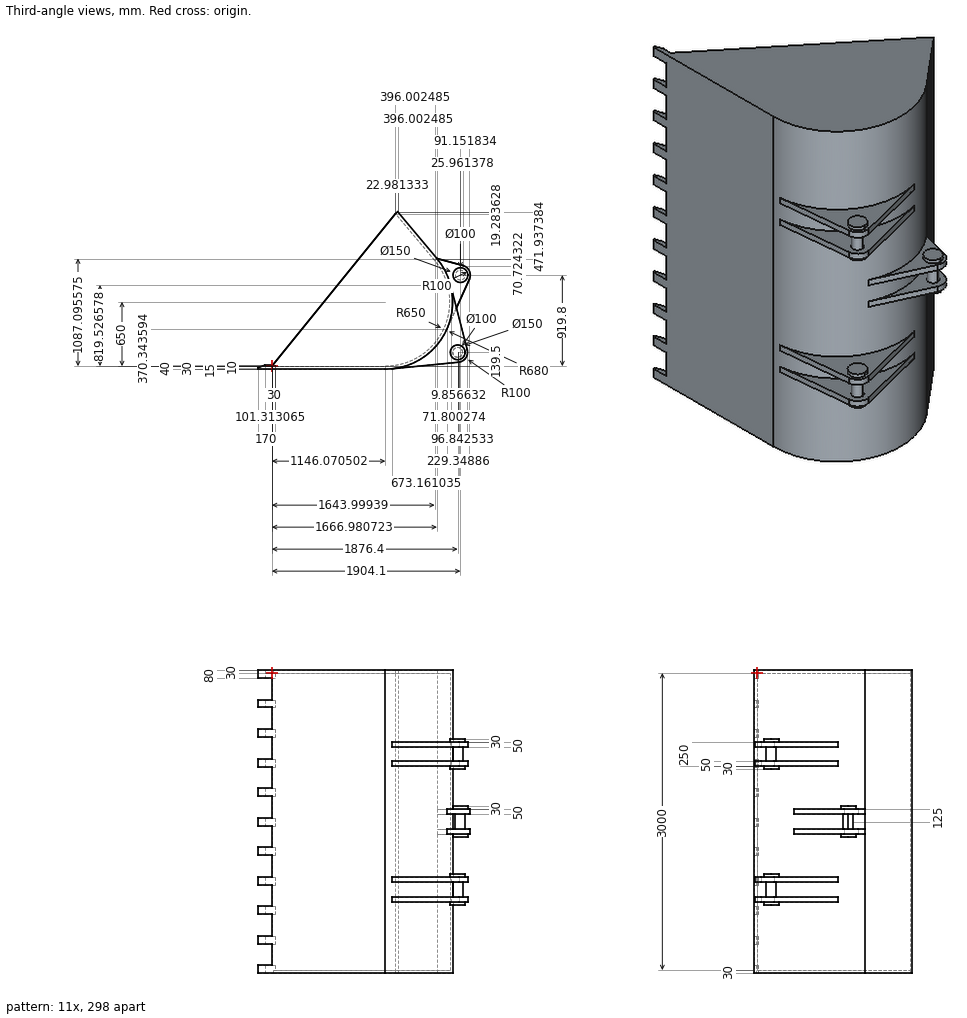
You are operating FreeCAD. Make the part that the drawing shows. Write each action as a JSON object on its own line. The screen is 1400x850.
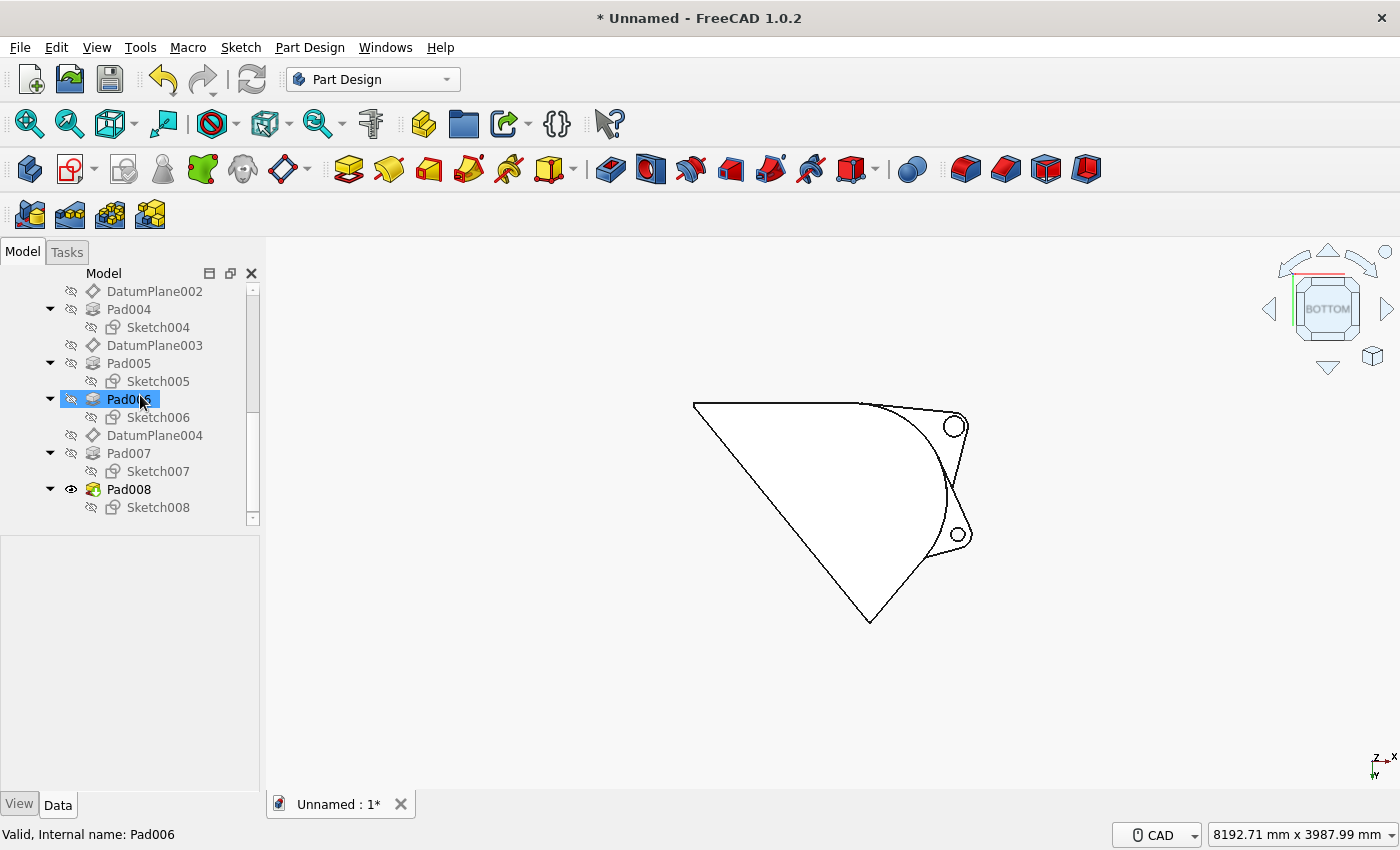
{"action": "scroll", "coordinate": [140, 395], "scroll_direction": "up", "scroll_amount": 15}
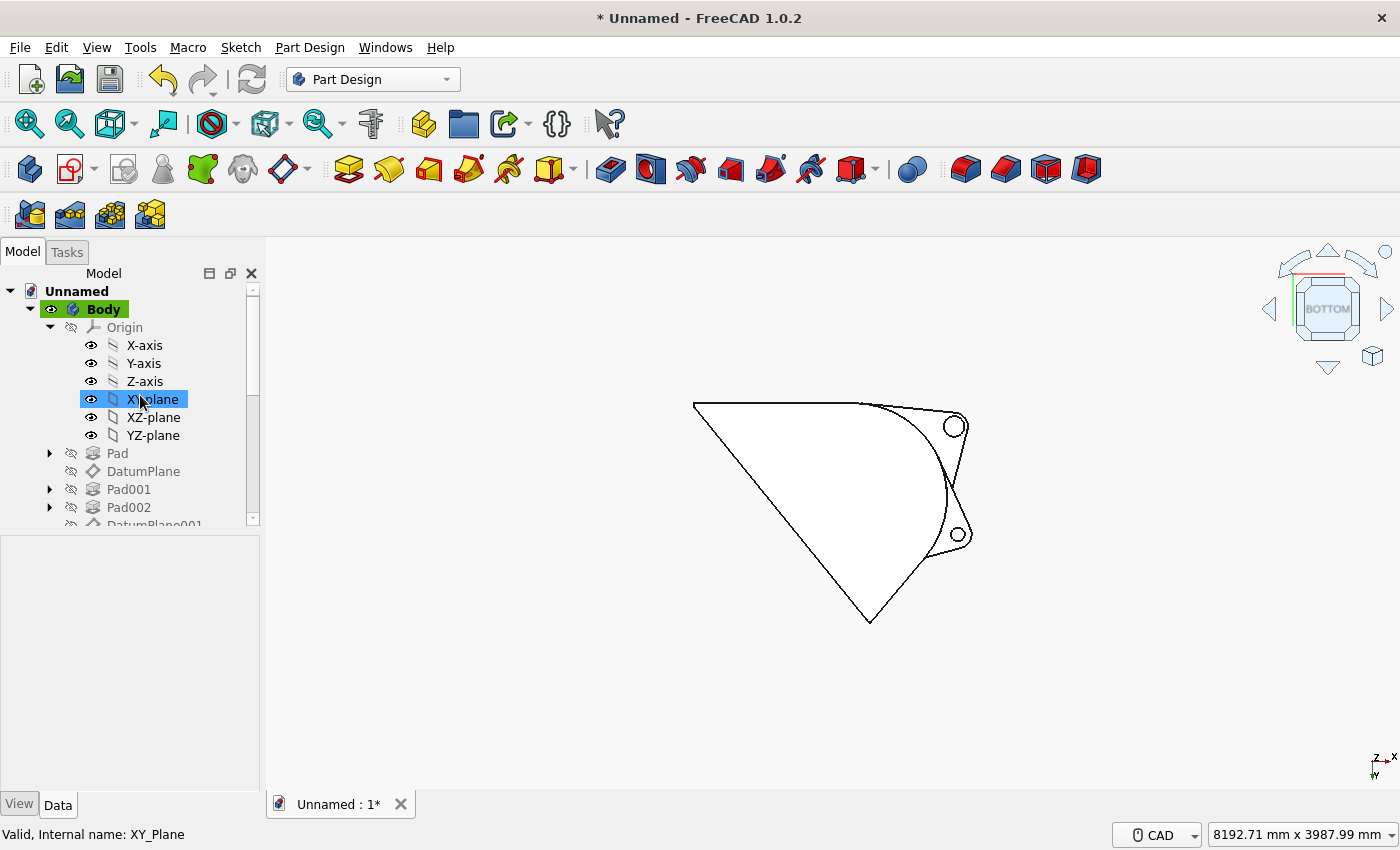
{"action": "left_click", "coordinate": [136, 399]}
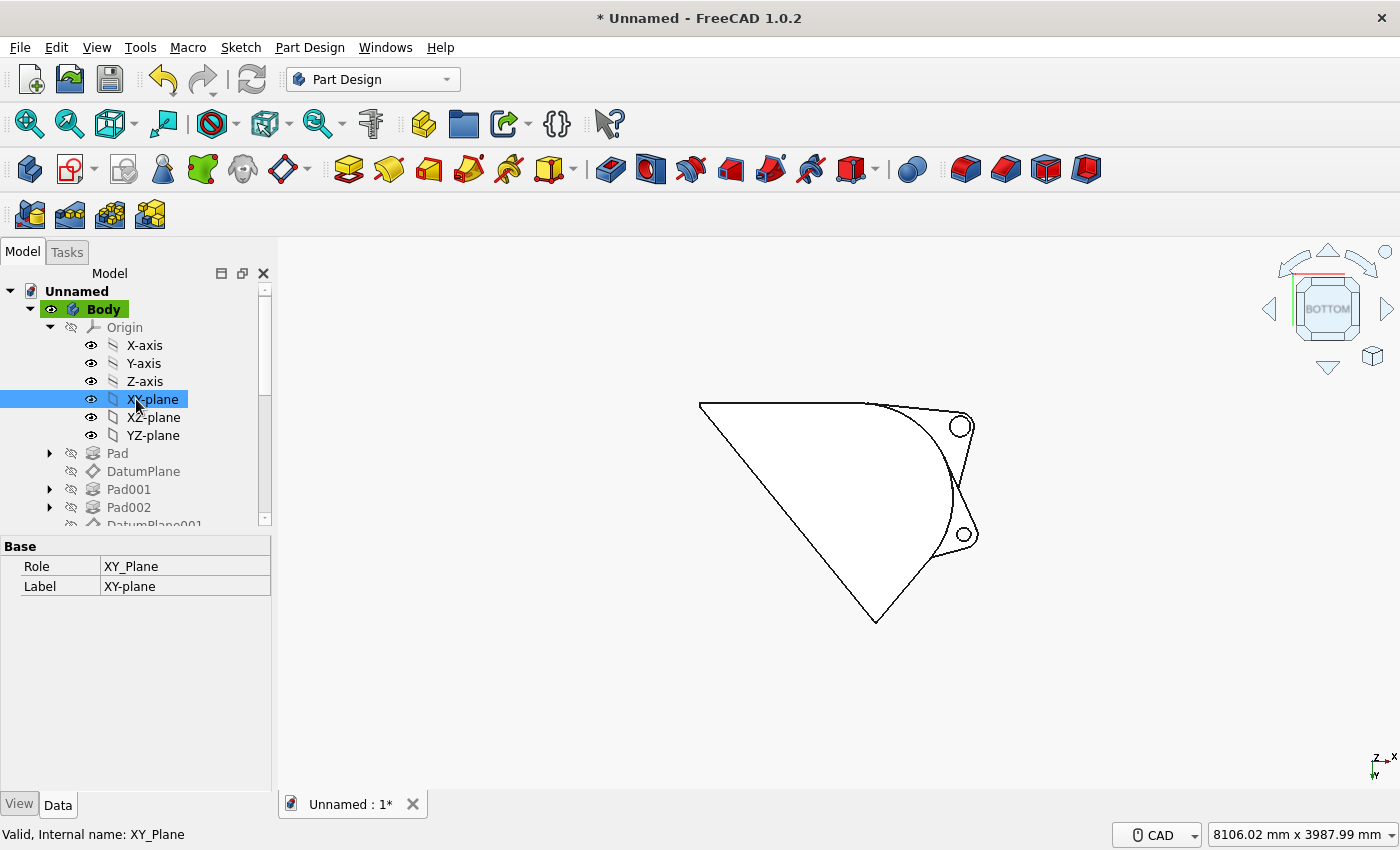
{"action": "left_click", "coordinate": [284, 170]}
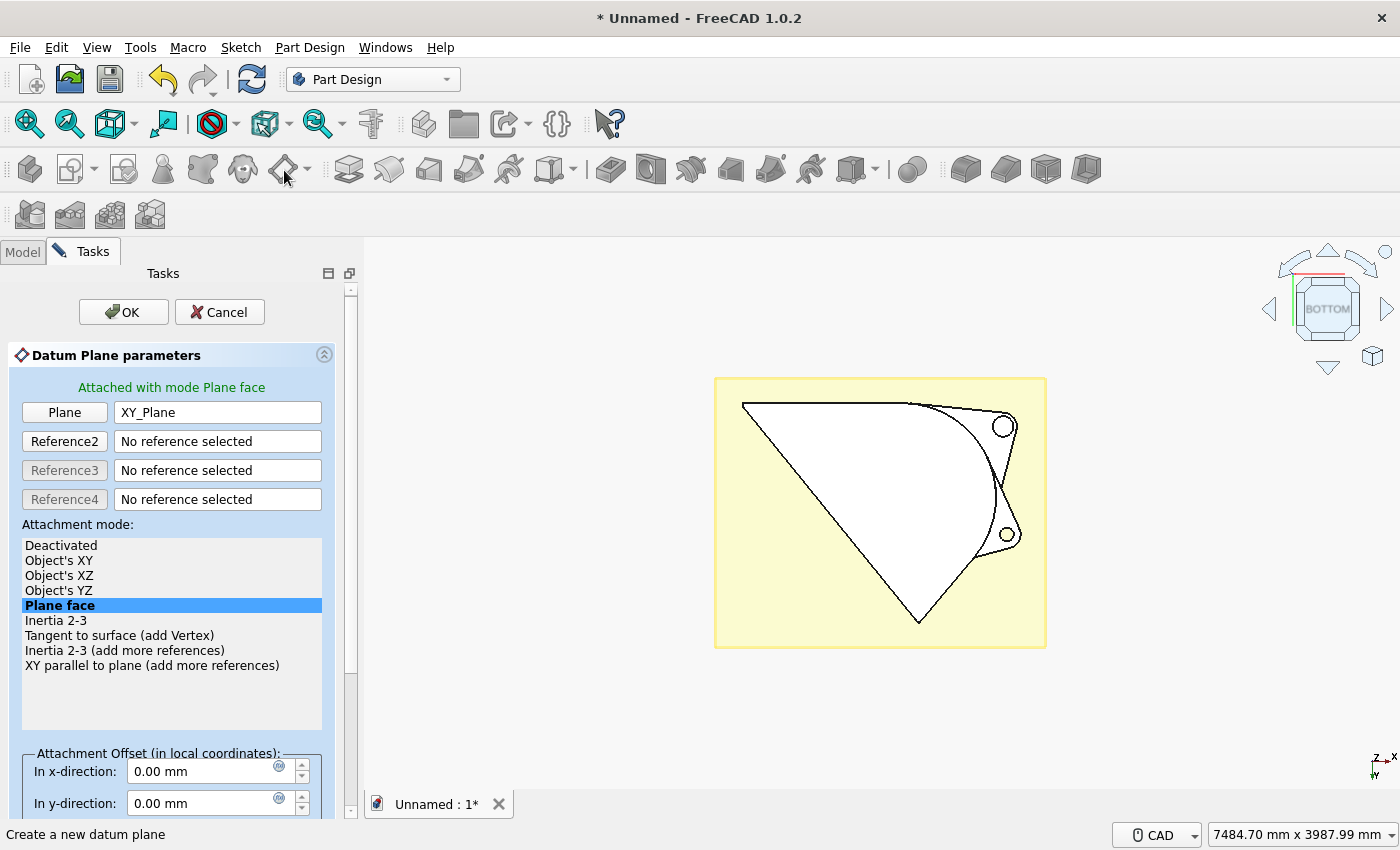
{"action": "scroll", "coordinate": [351, 550], "scroll_direction": "down", "scroll_amount": 2}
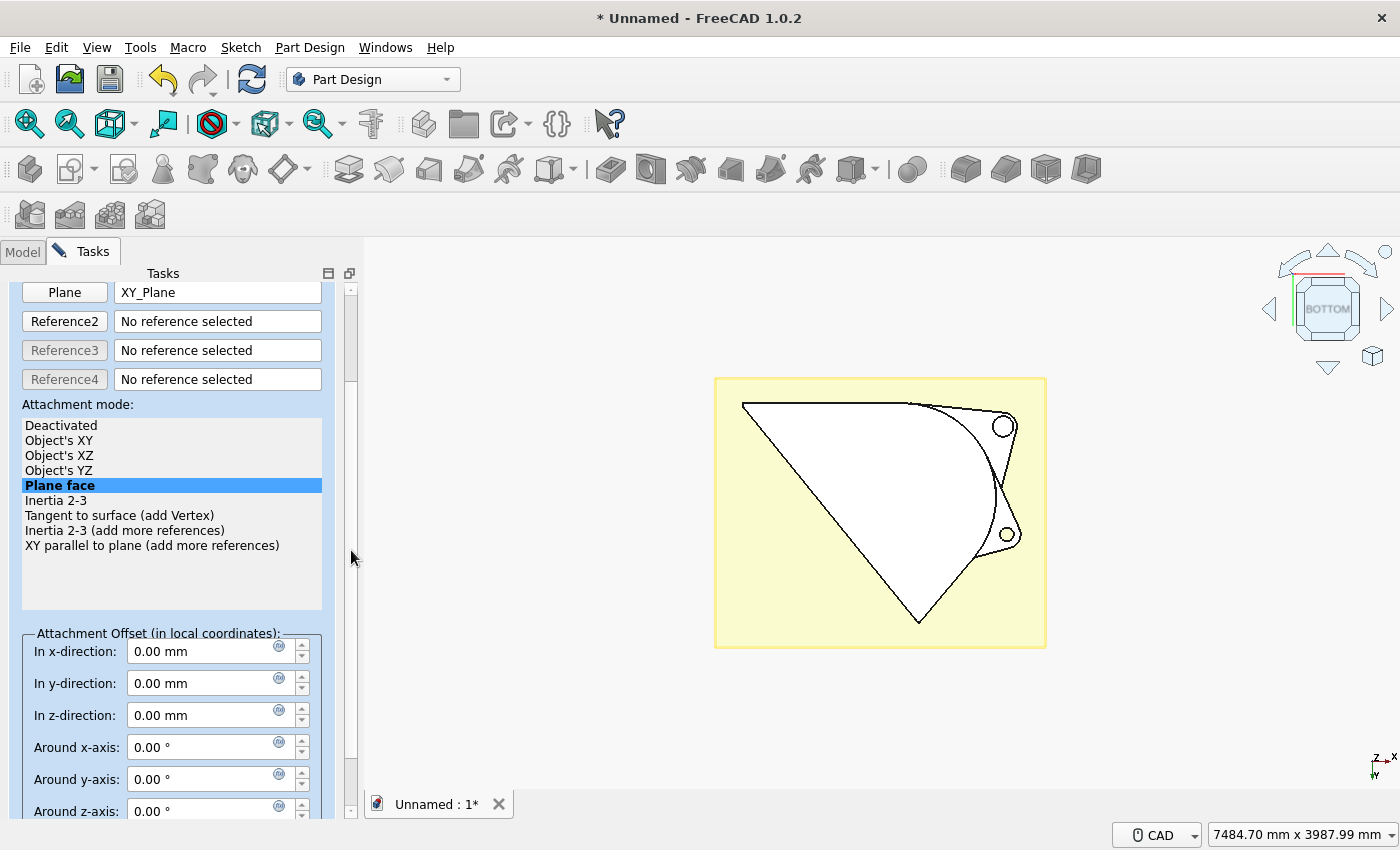
{"action": "triple_click", "coordinate": [210, 715]}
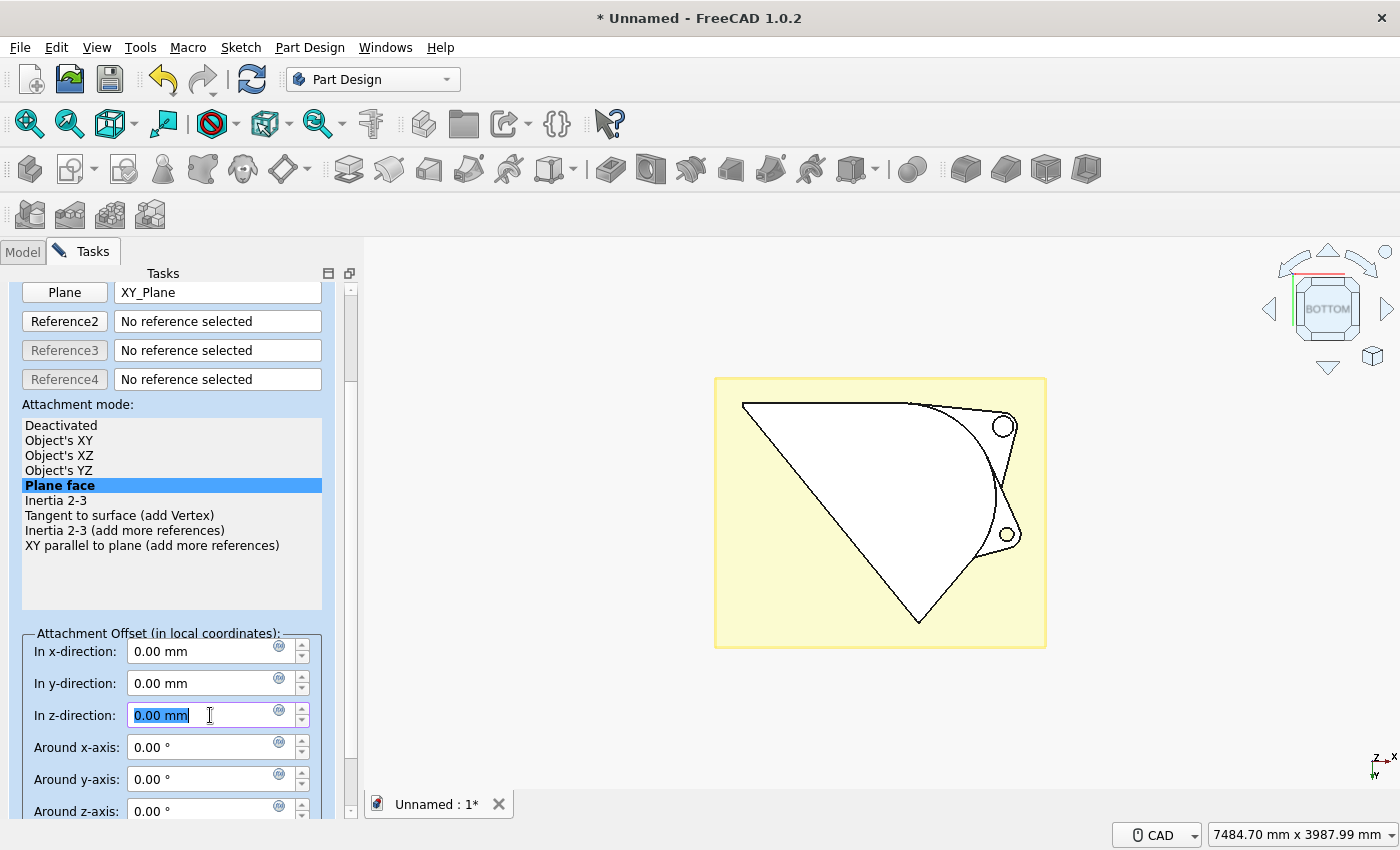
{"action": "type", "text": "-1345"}
{"action": "key", "text": "Tab"}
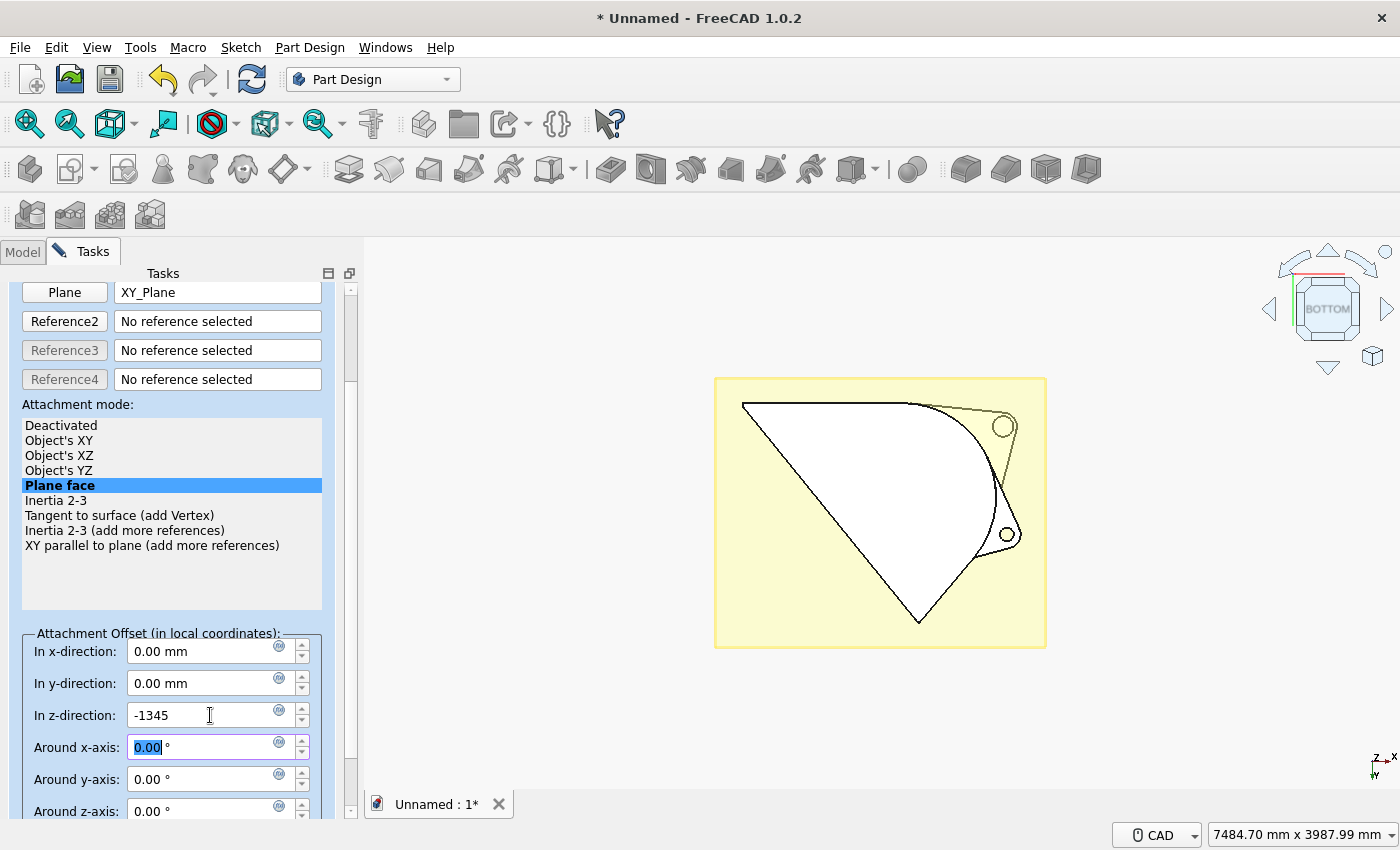
{"action": "scroll", "coordinate": [351, 550], "scroll_direction": "up", "scroll_amount": 3}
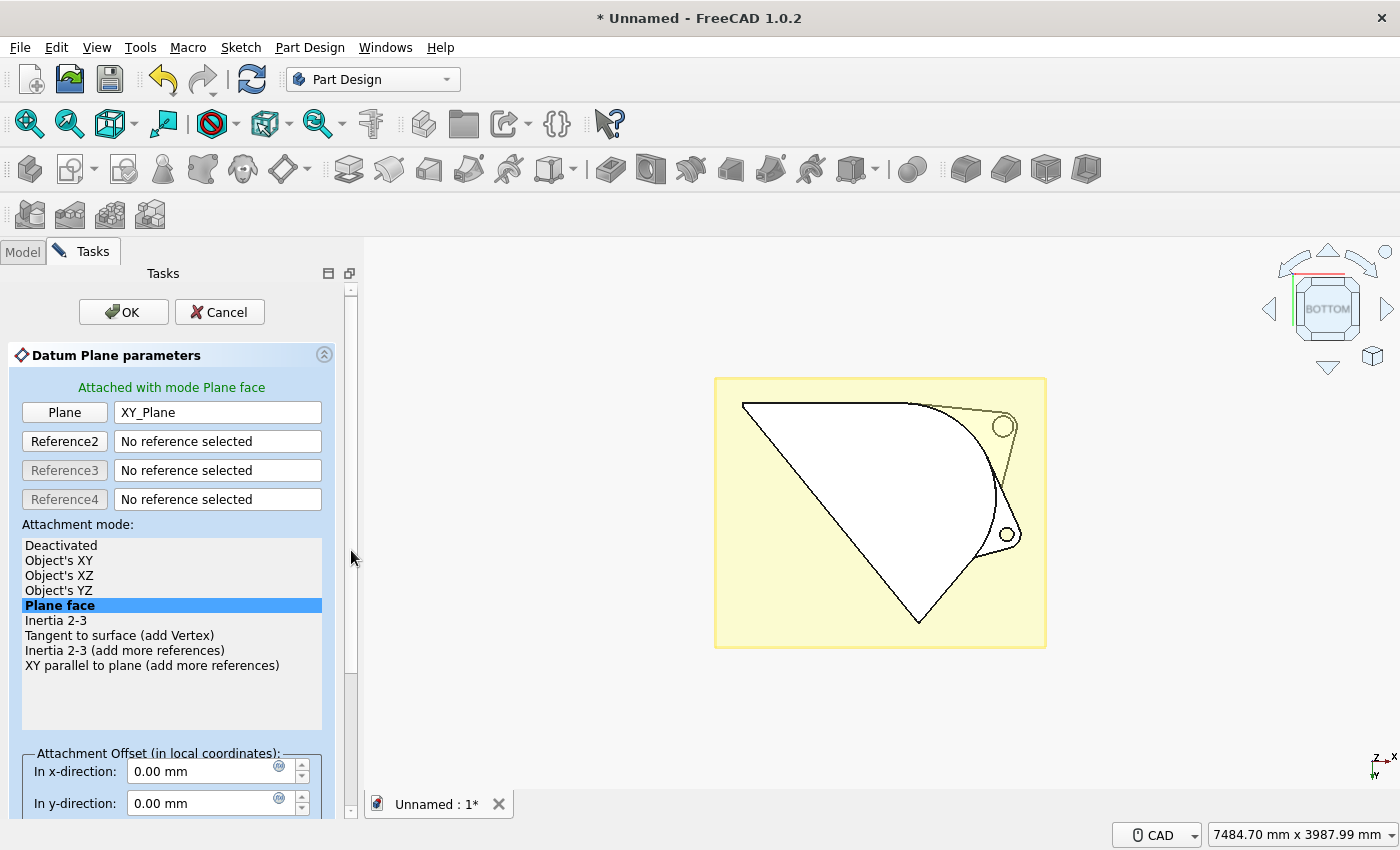
{"action": "left_click", "coordinate": [124, 312]}